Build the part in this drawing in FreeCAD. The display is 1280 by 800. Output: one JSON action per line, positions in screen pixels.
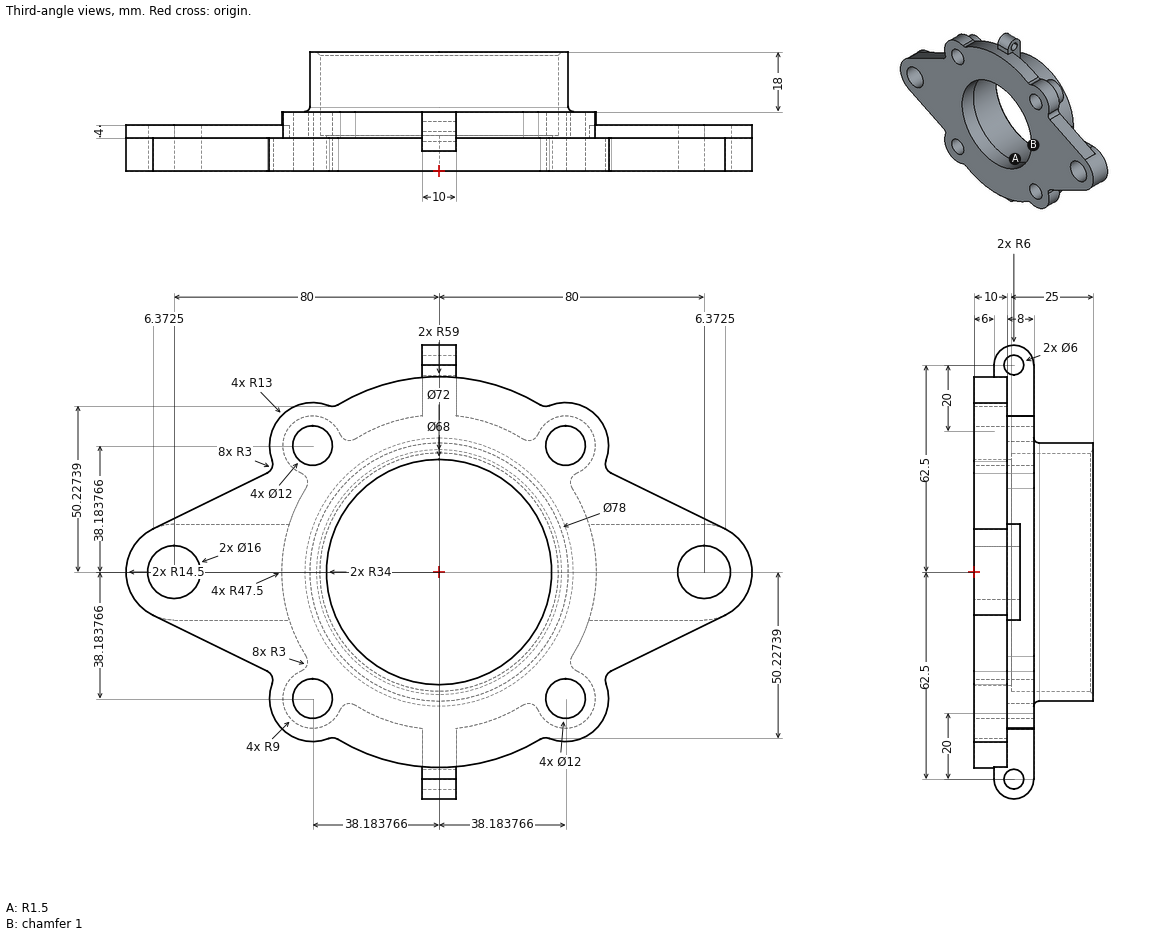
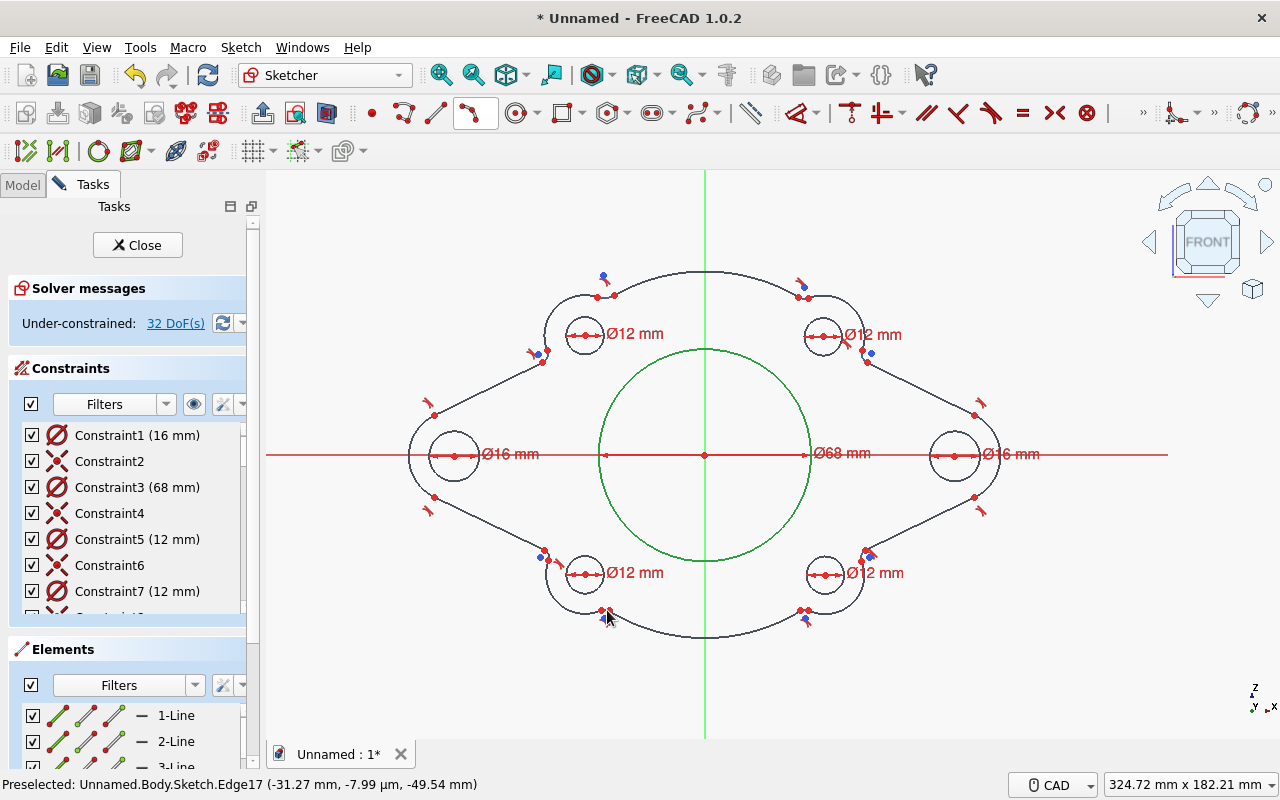
{"action": "scroll", "coordinate": [549, 557], "scroll_direction": "up", "scroll_amount": 7}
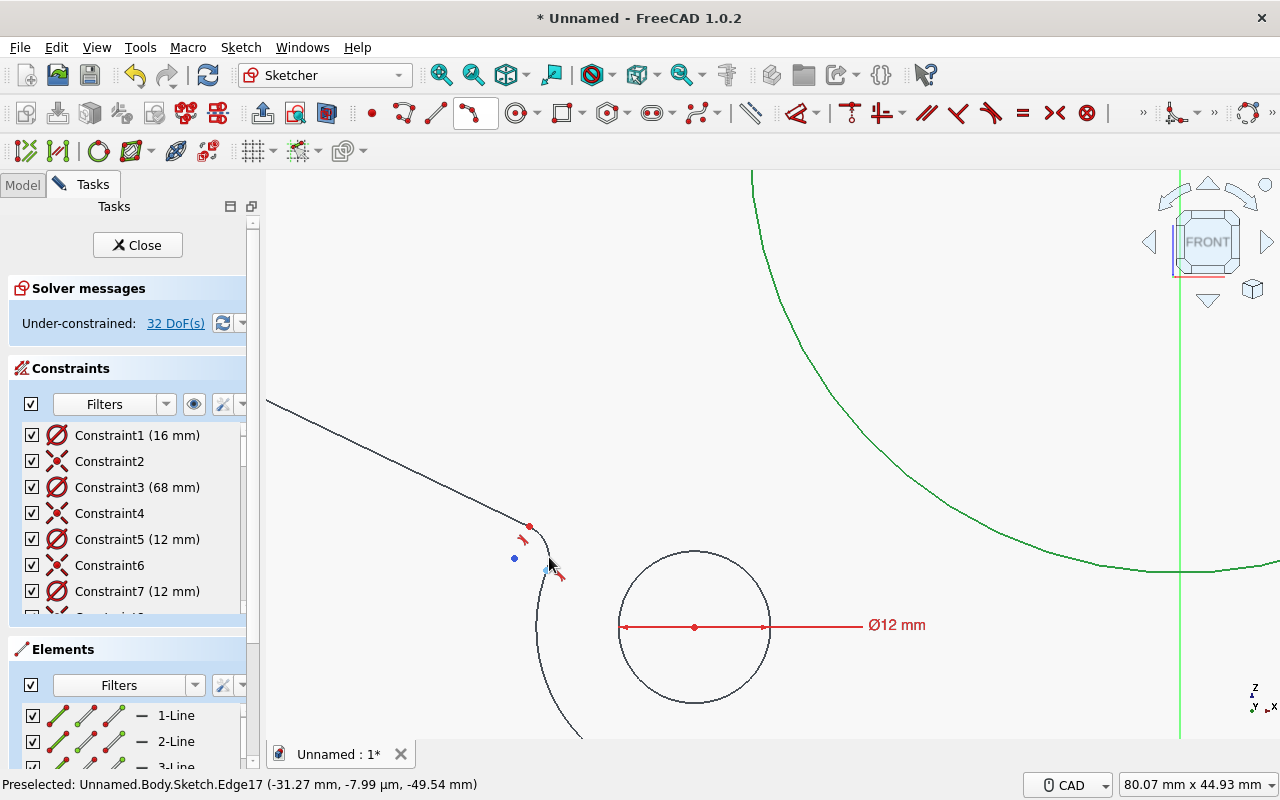
{"action": "left_click", "coordinate": [549, 555]}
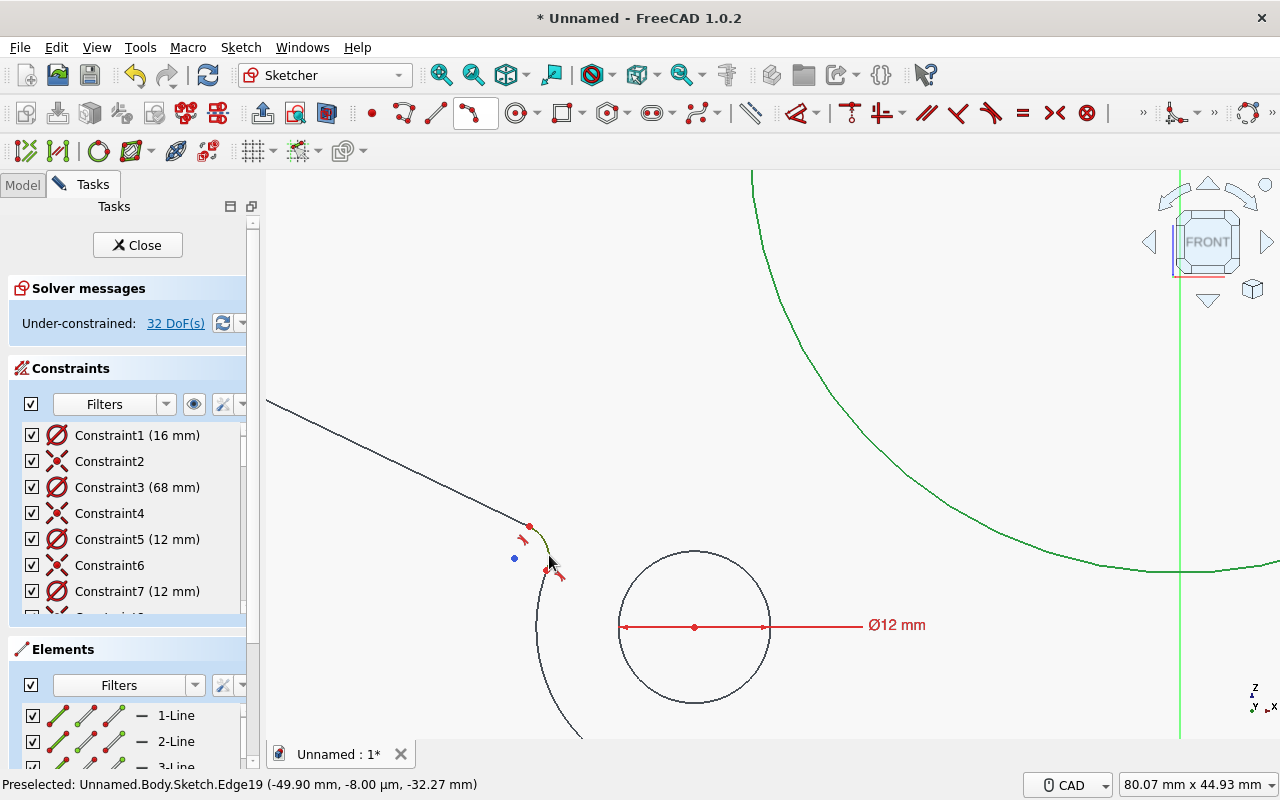
{"action": "left_click", "coordinate": [1024, 114]}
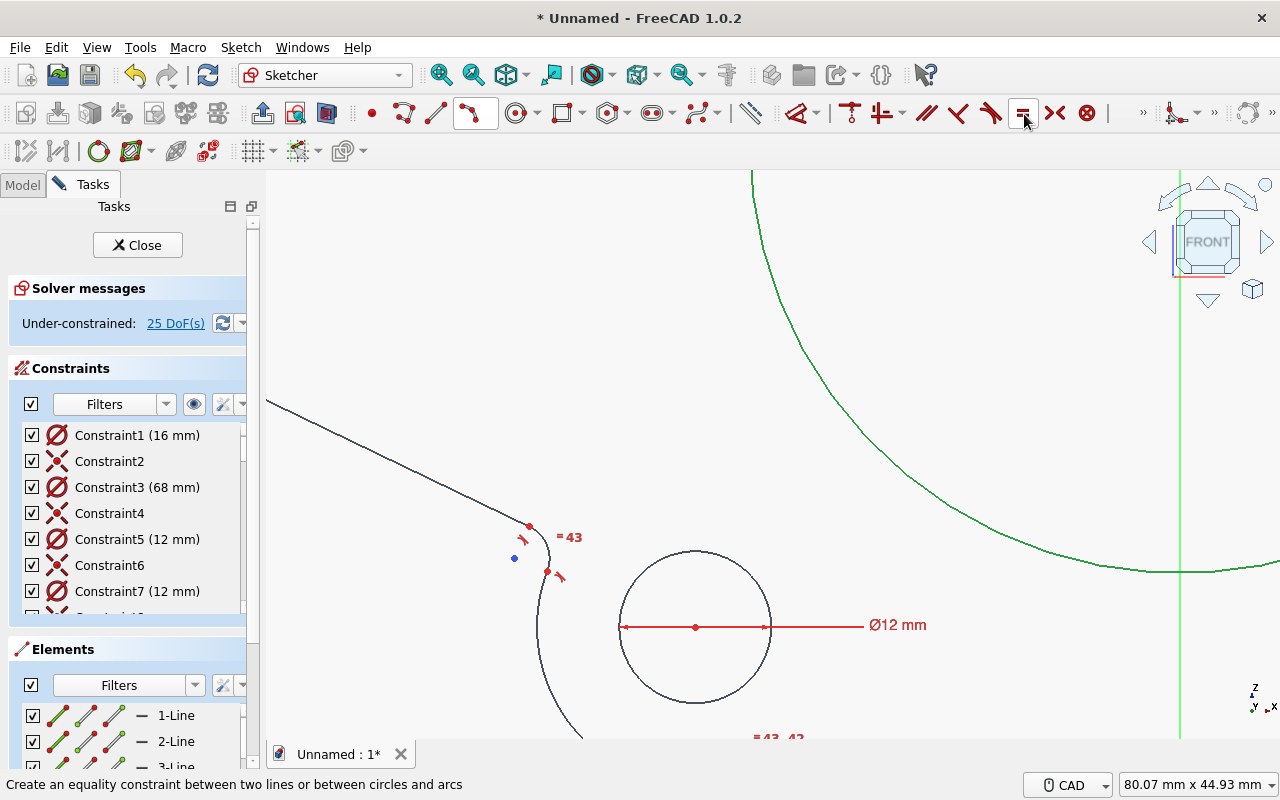
{"action": "scroll", "coordinate": [549, 557], "scroll_direction": "down", "scroll_amount": 7}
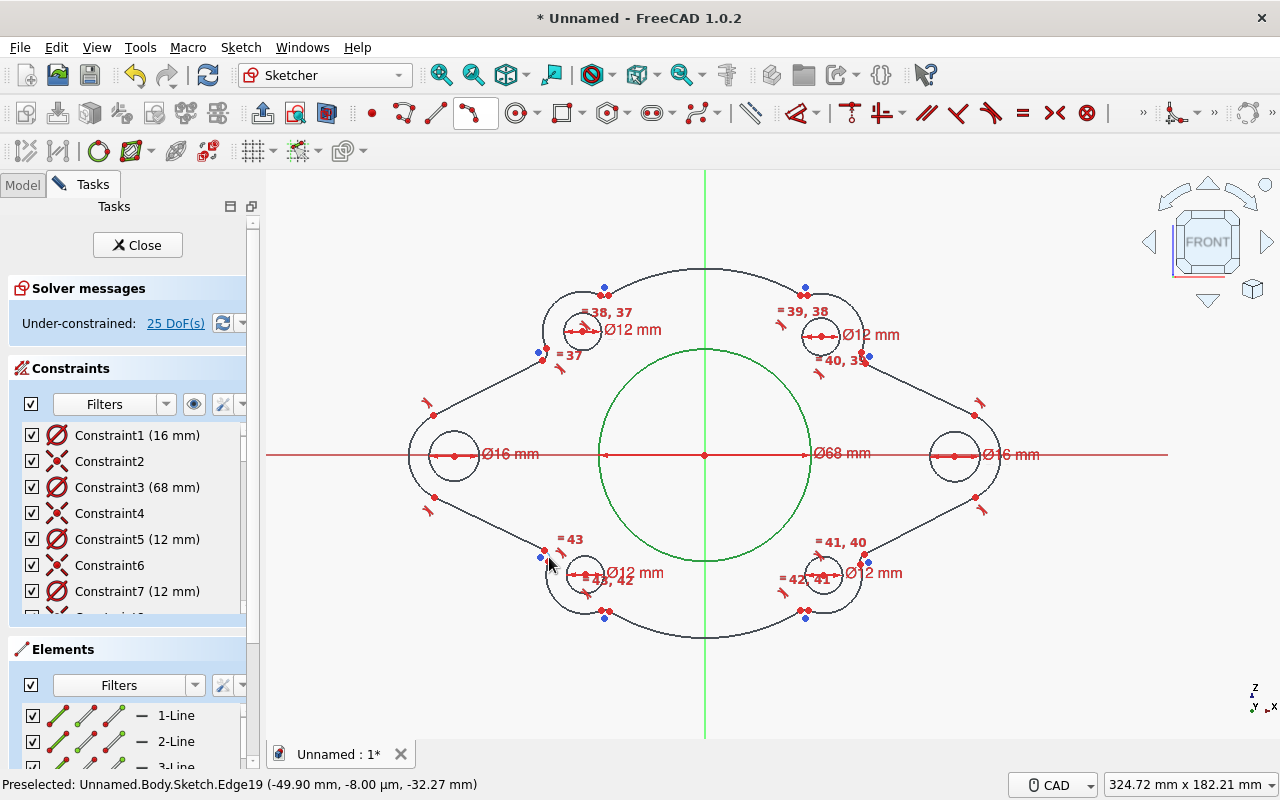
{"action": "left_click", "coordinate": [572, 293]}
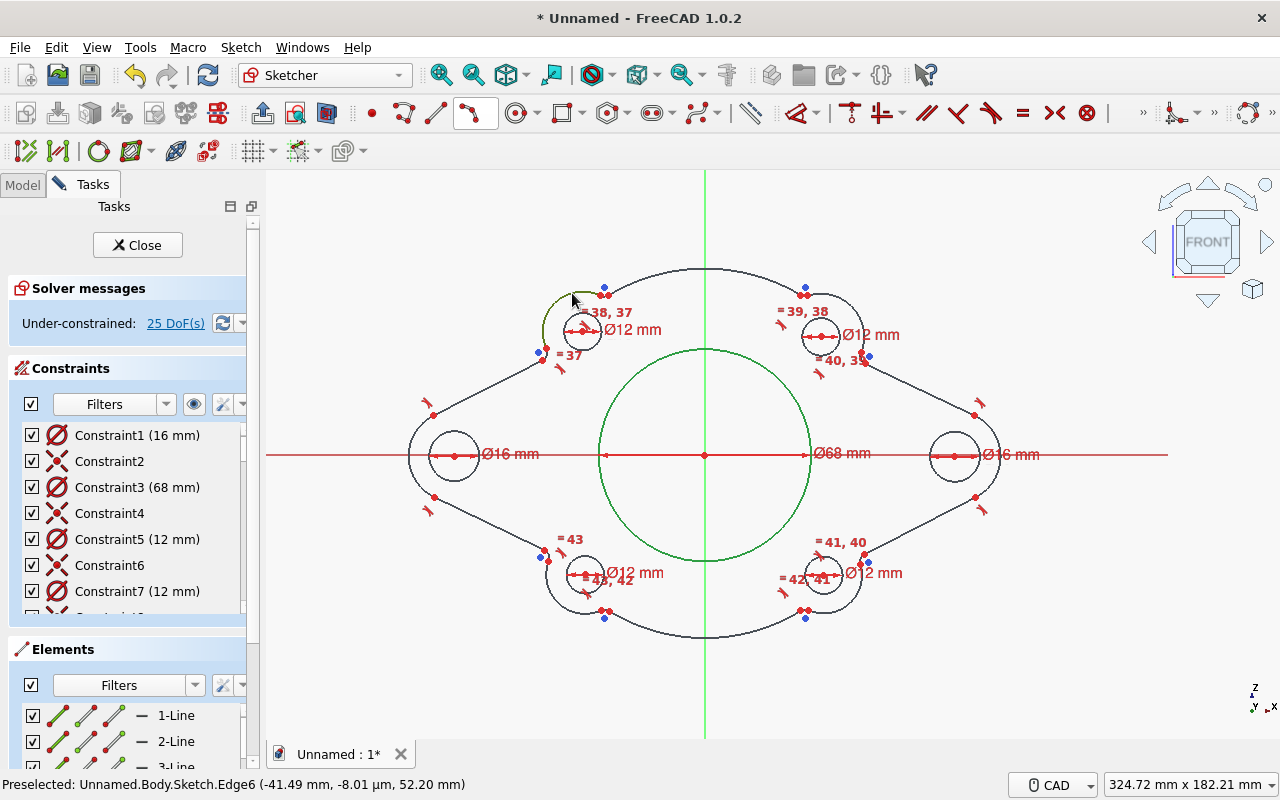
{"action": "left_click", "coordinate": [862, 324]}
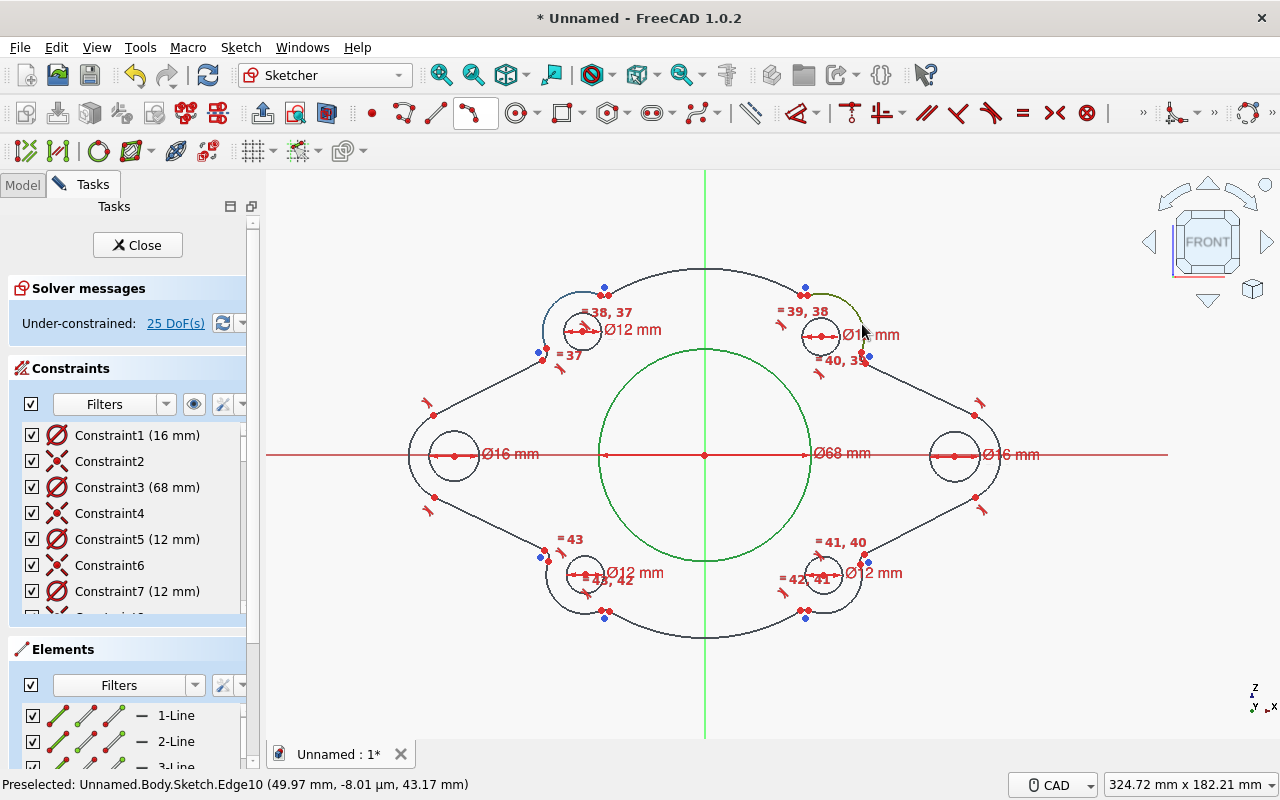
{"action": "left_click", "coordinate": [834, 612]}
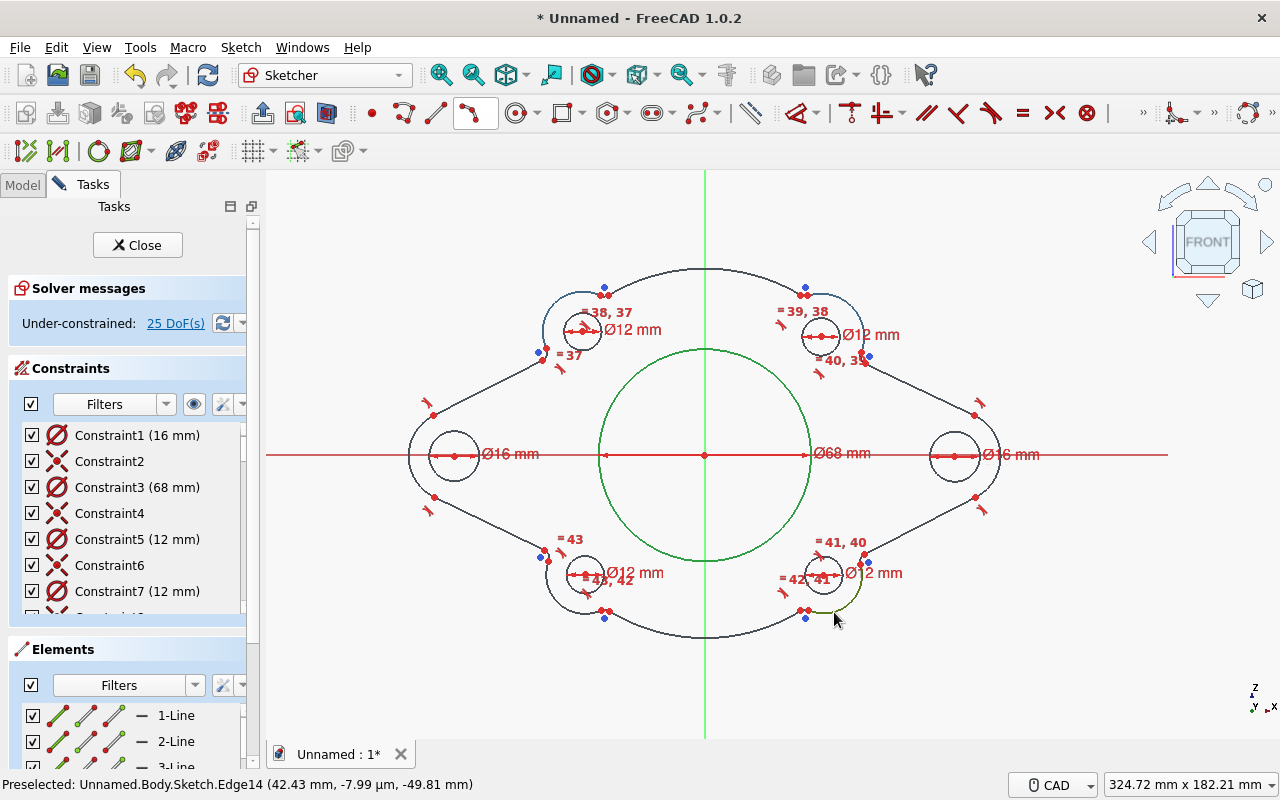
{"action": "left_click", "coordinate": [549, 588]}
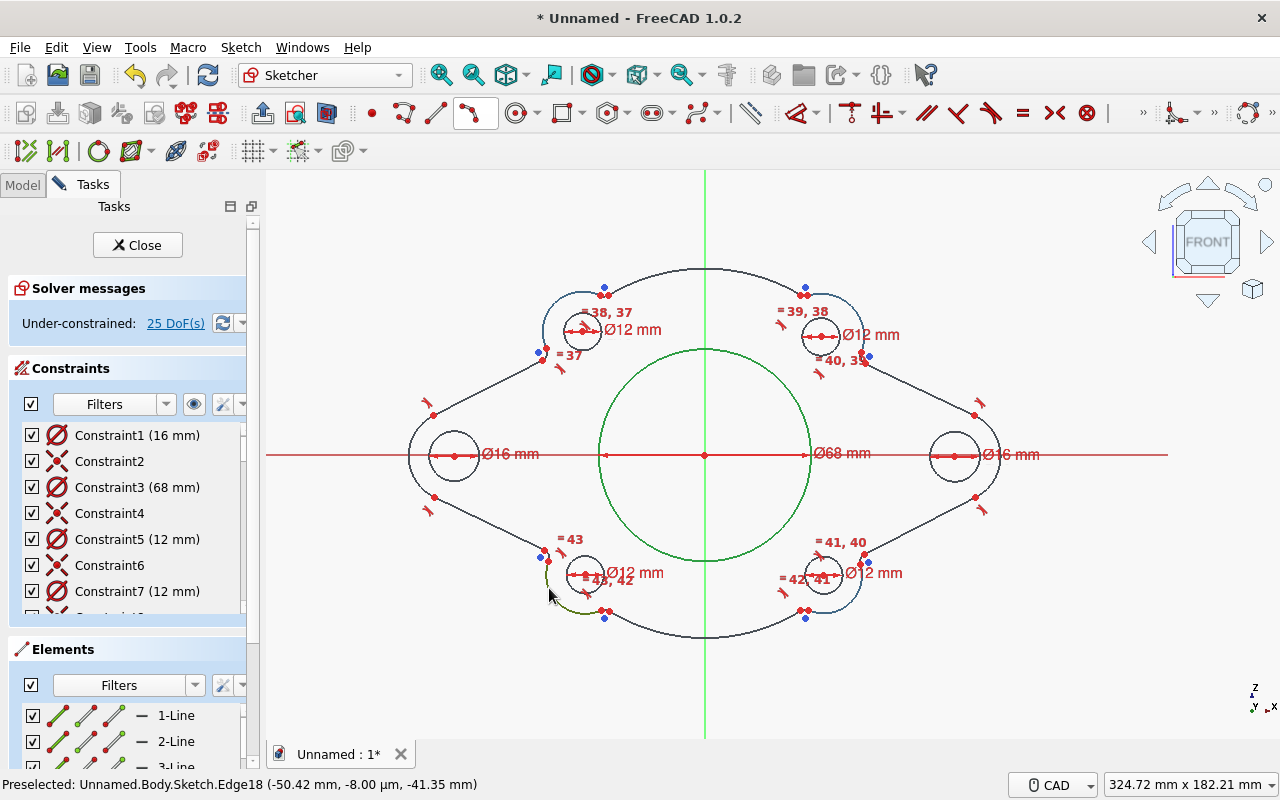
{"action": "left_click", "coordinate": [1024, 114]}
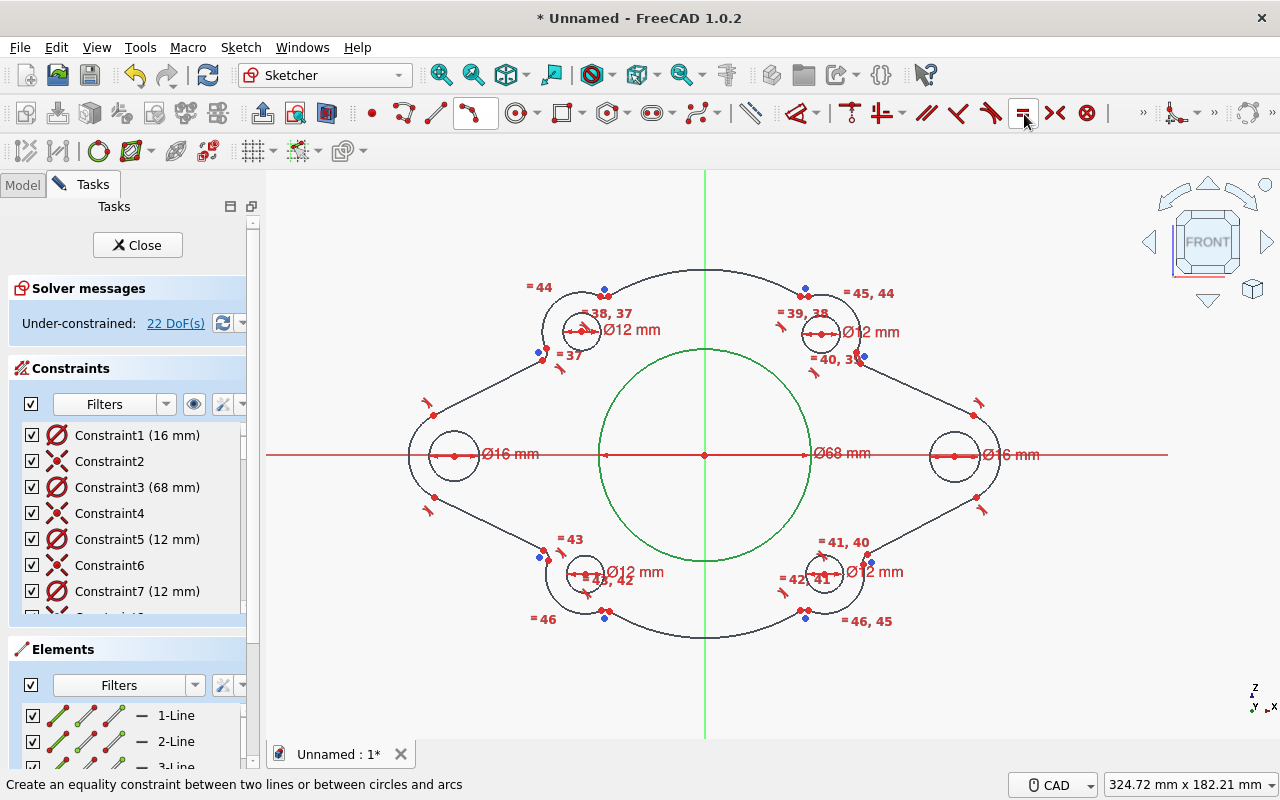
{"action": "left_click", "coordinate": [745, 274]}